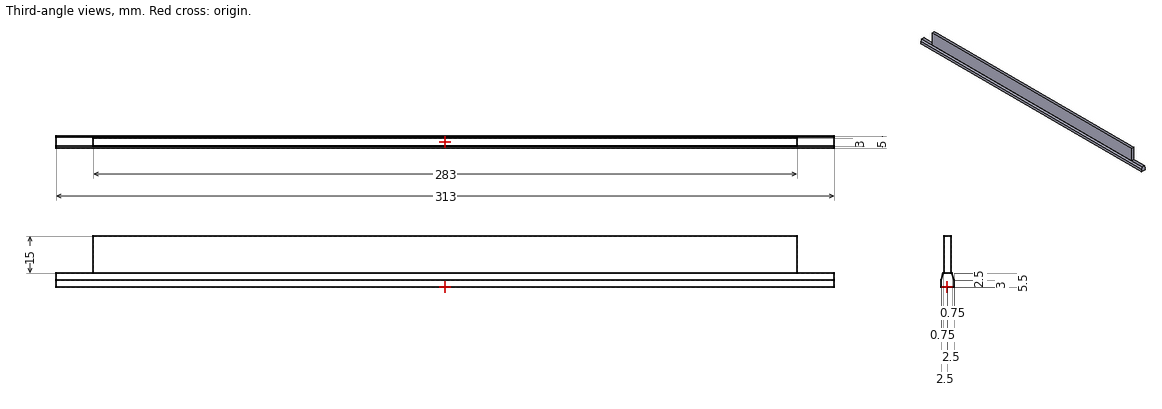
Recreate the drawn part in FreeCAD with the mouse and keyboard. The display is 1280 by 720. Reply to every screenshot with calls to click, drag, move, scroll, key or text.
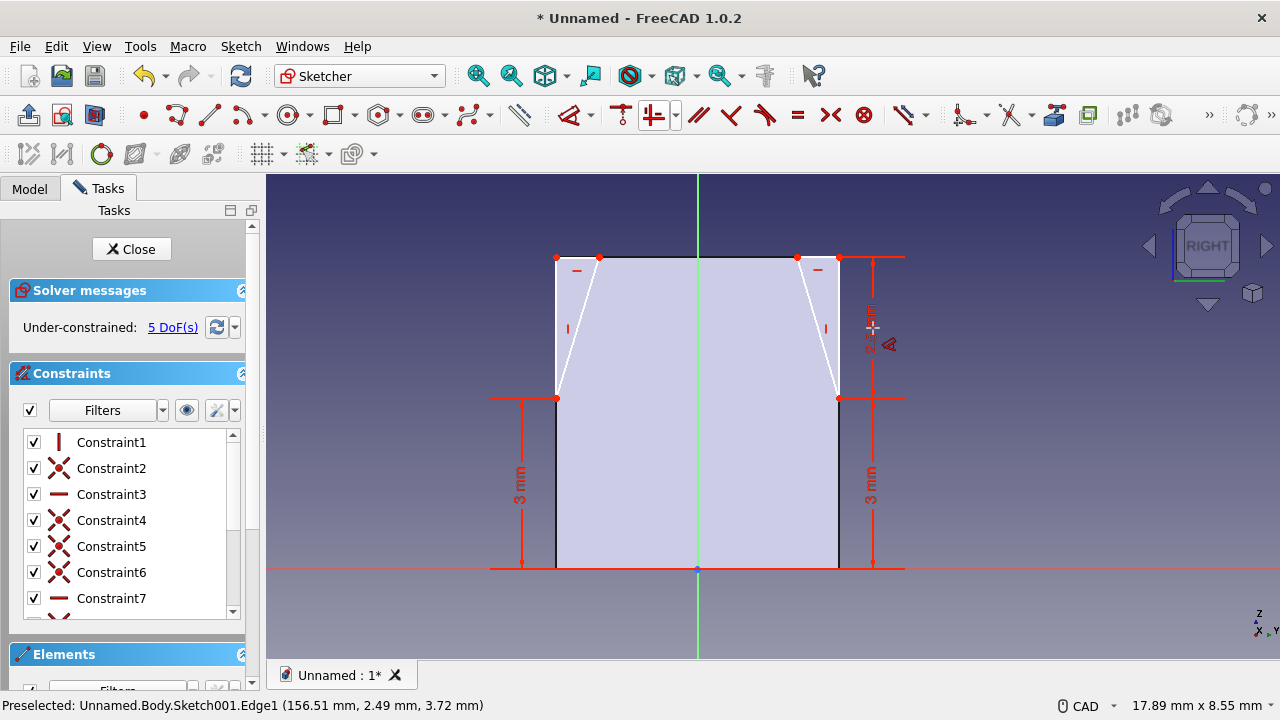
click(556, 300)
click(522, 328)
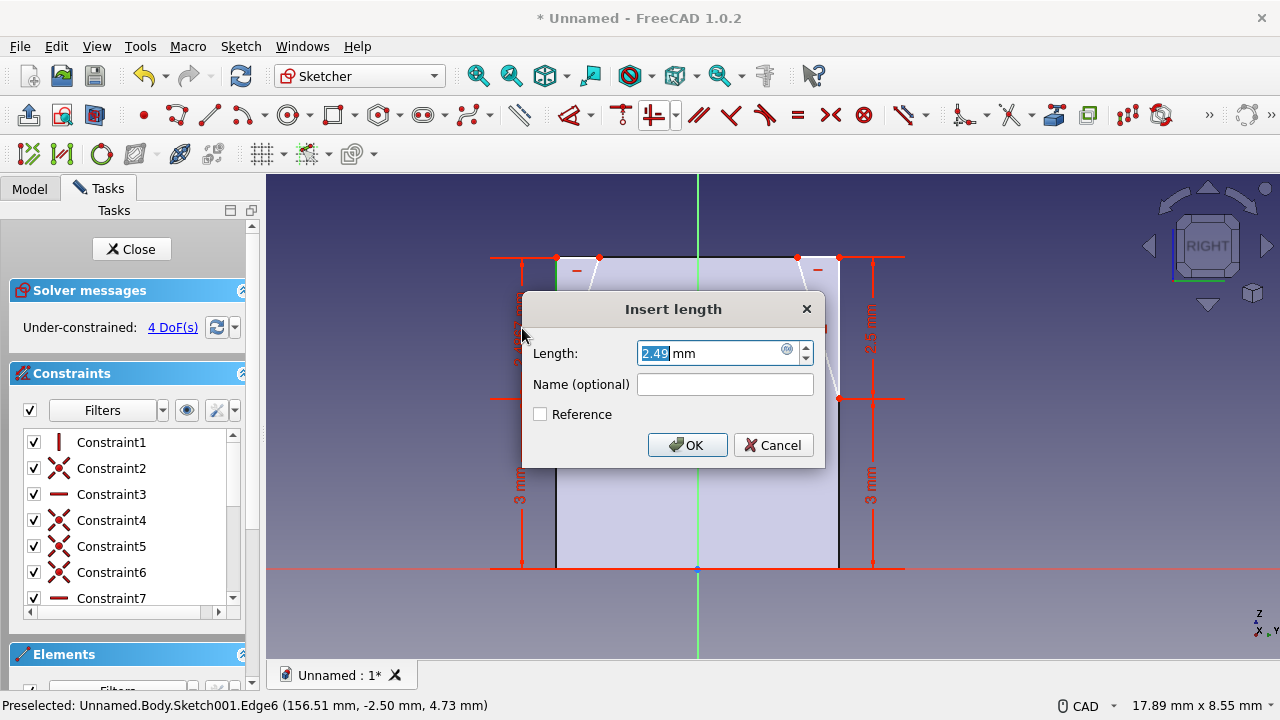
text(2.5)
key(Return)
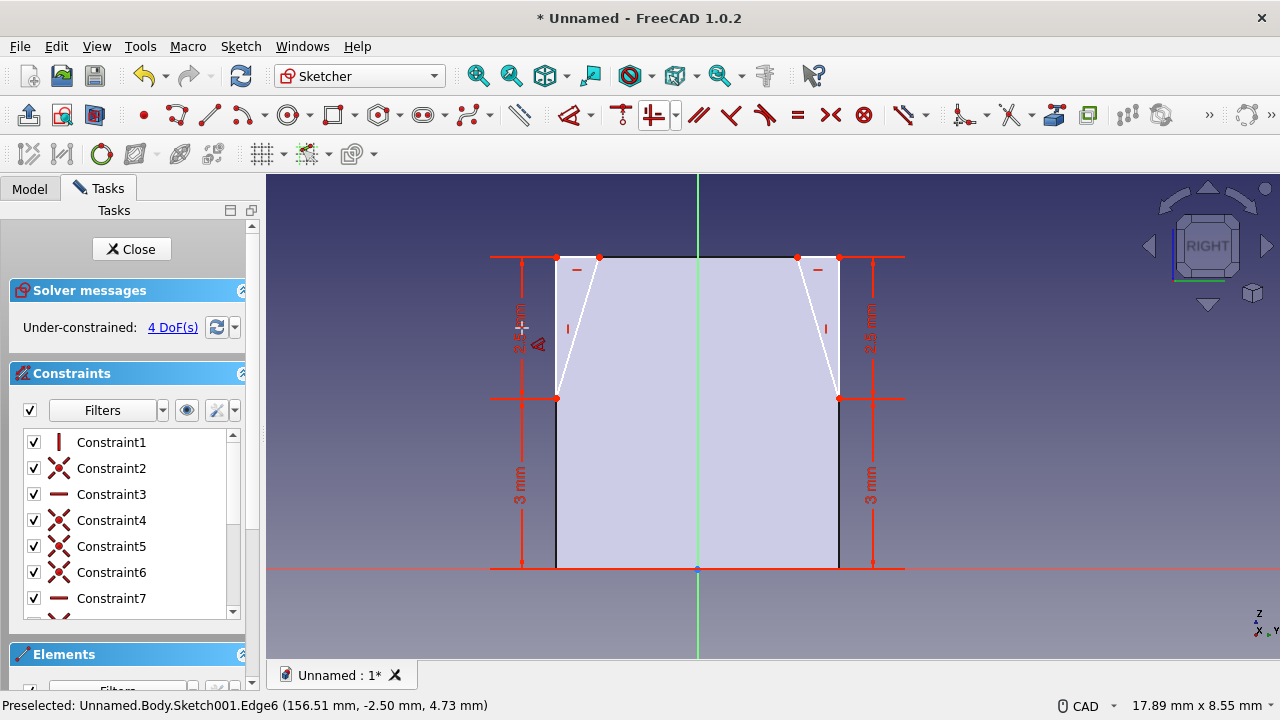
click(826, 257)
click(818, 223)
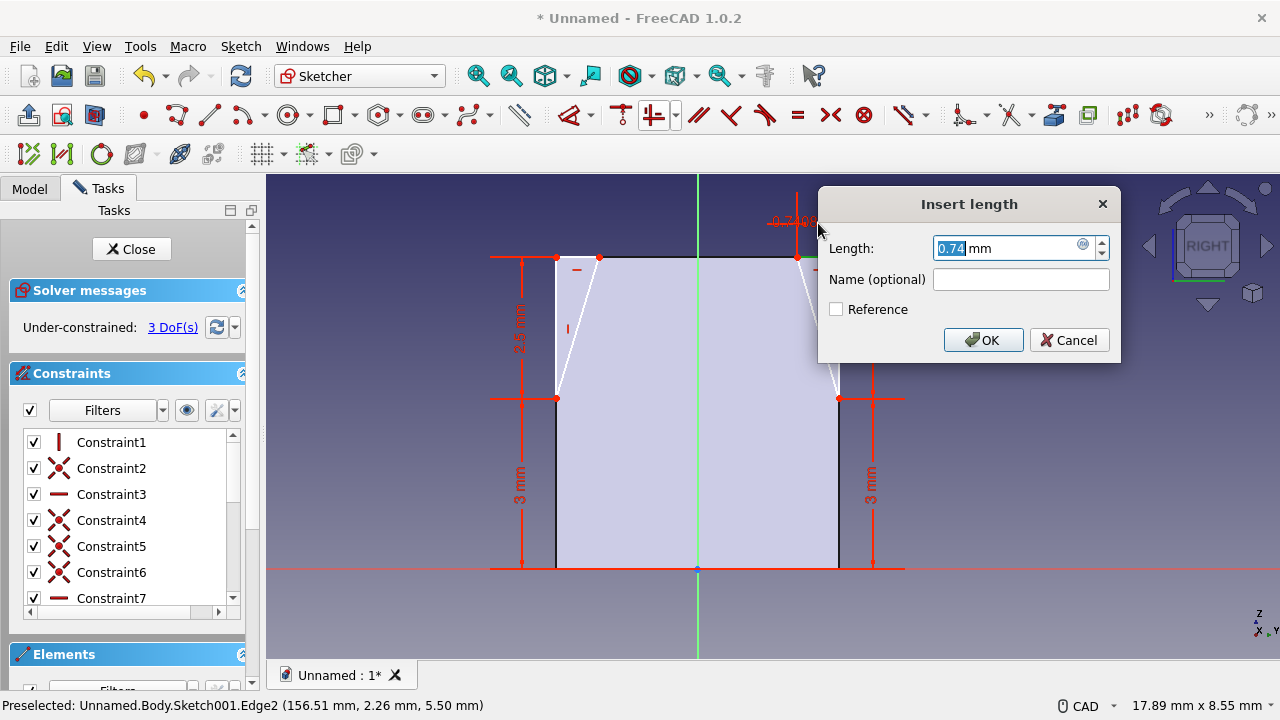
text(0.75)
key(Return)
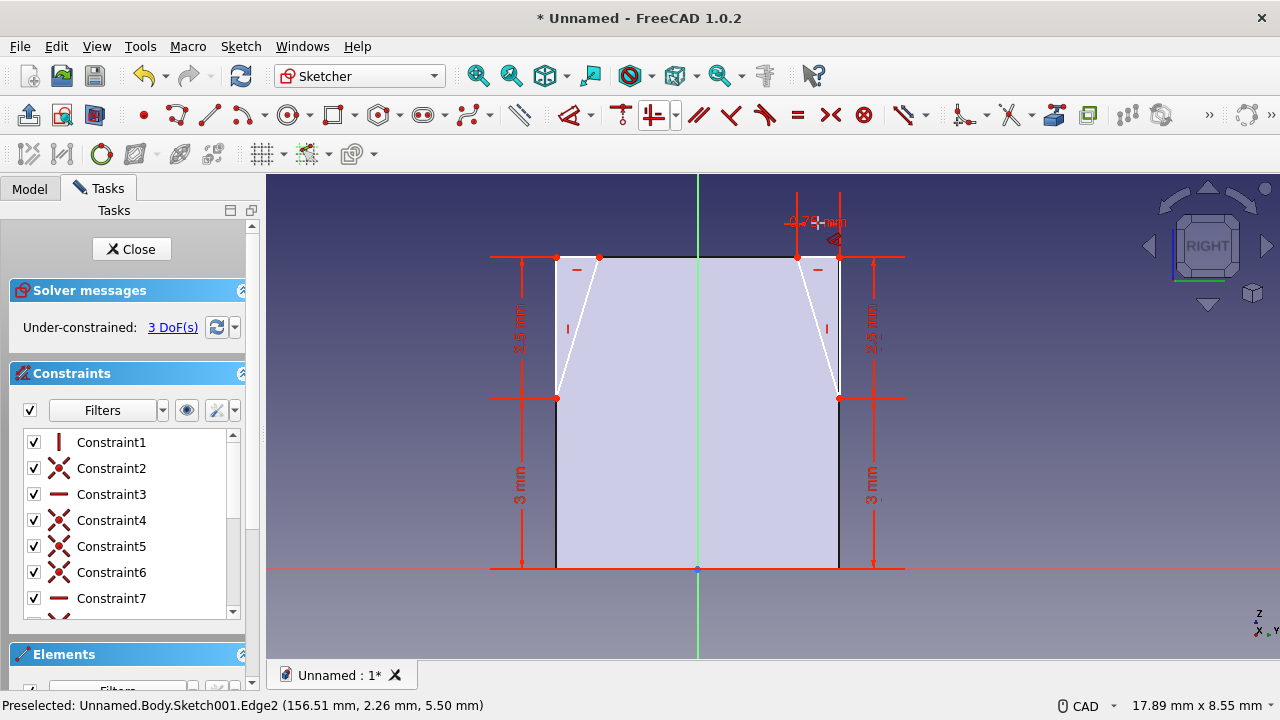
click(586, 257)
click(577, 223)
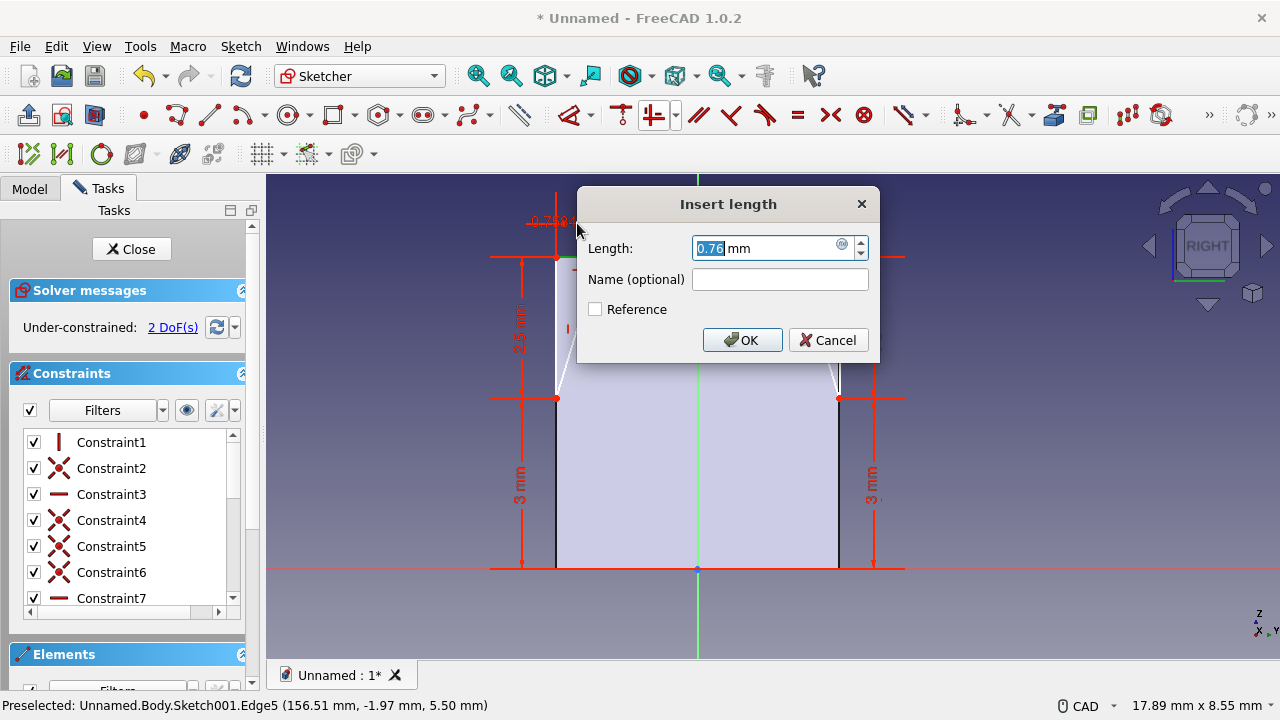
text(0.75)
key(Return)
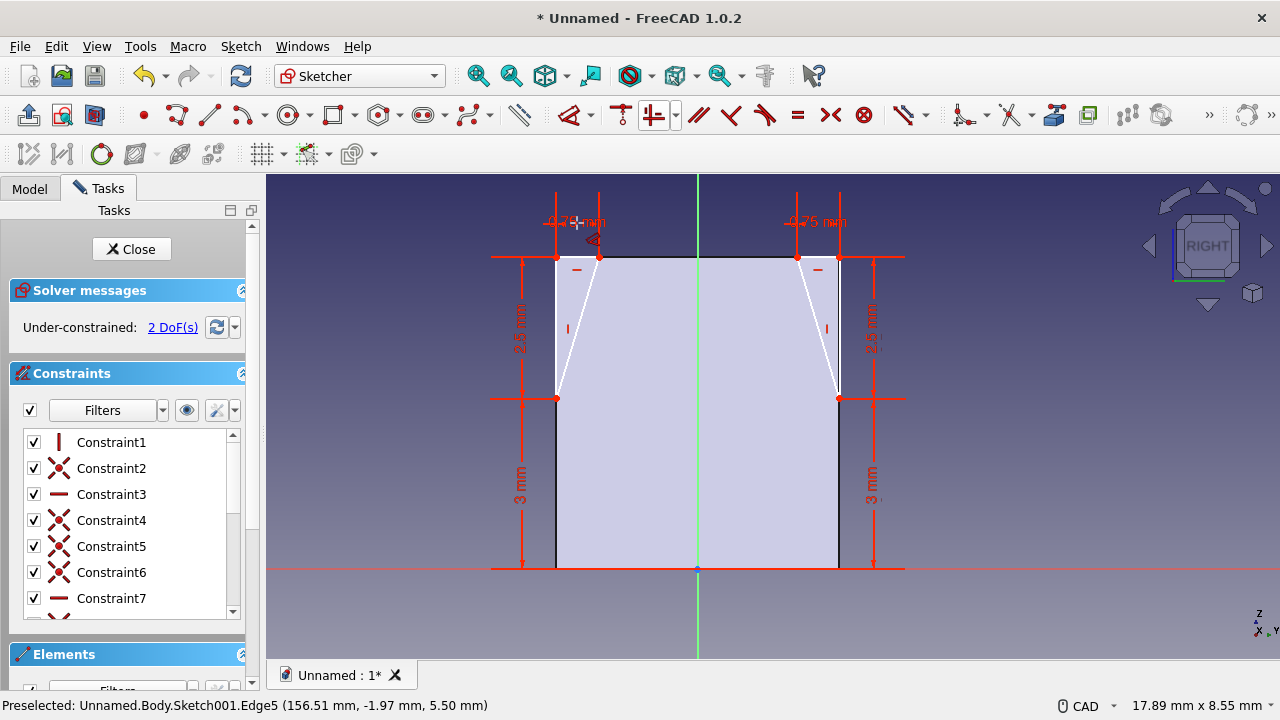
click(840, 399)
click(769, 603)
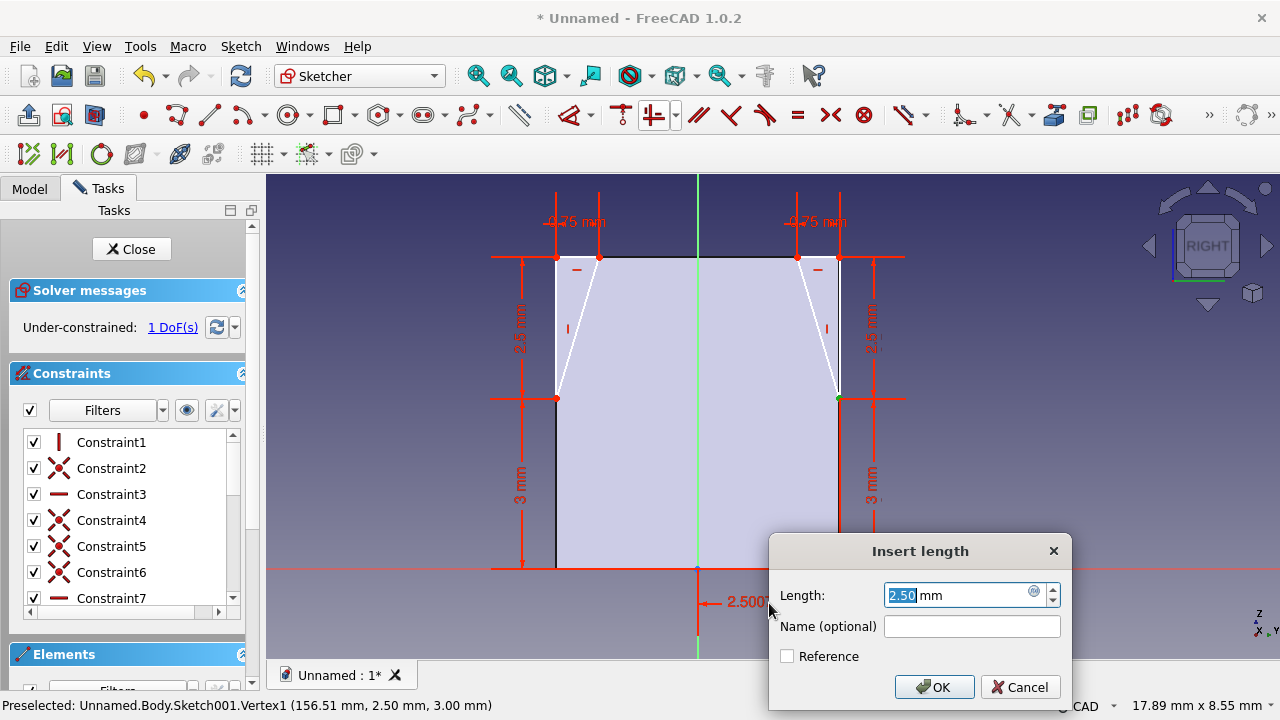
text(2.5)
key(Return)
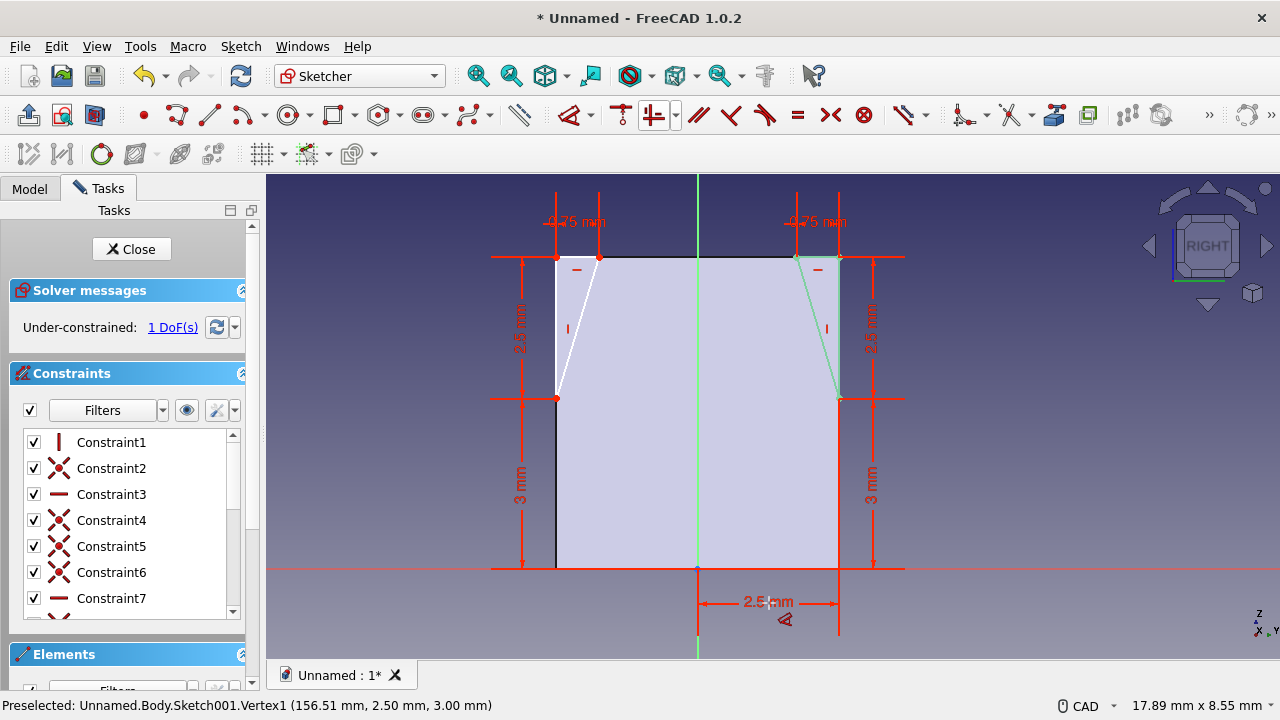
click(556, 399)
click(627, 603)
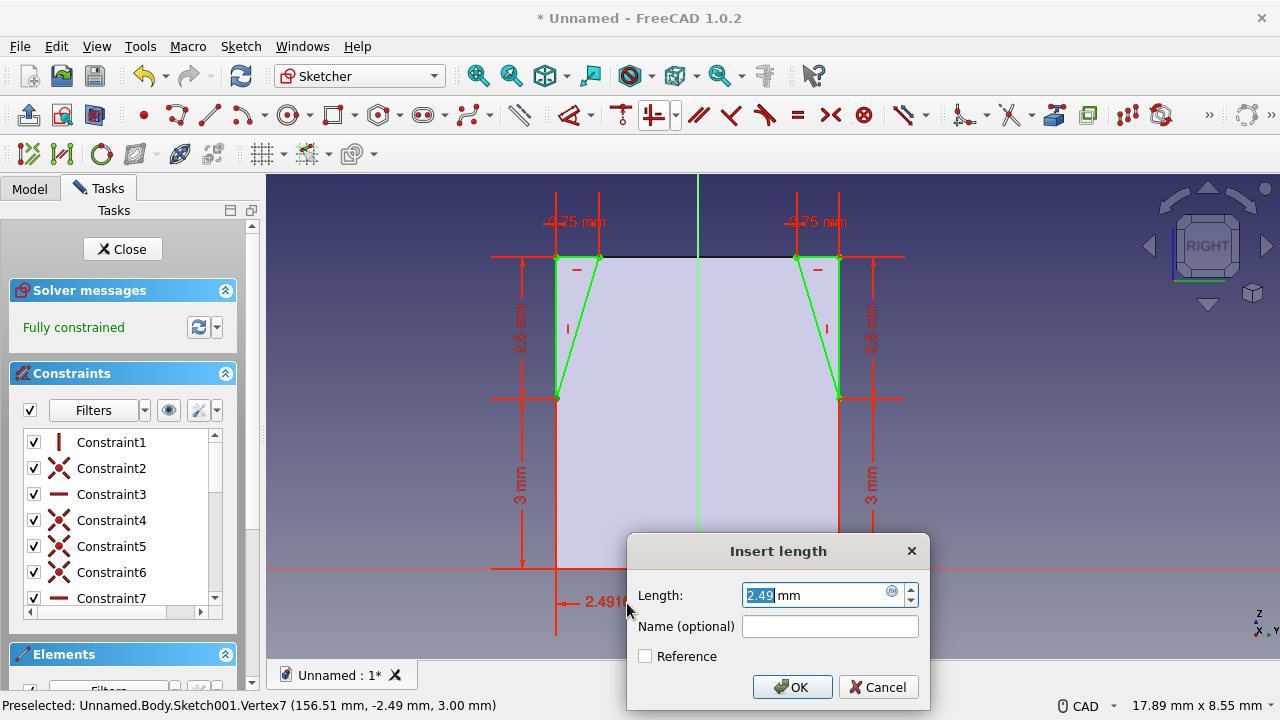
text(2.5)
key(Return)
key(Escape)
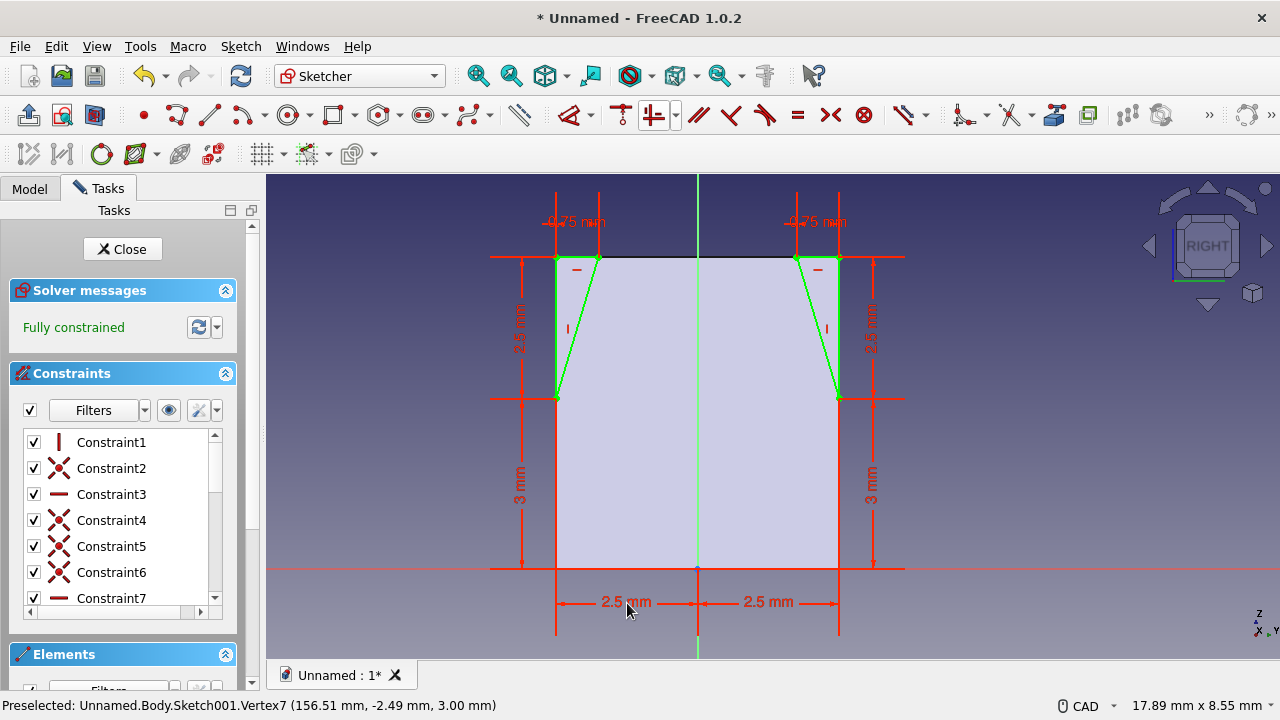
click(123, 249)